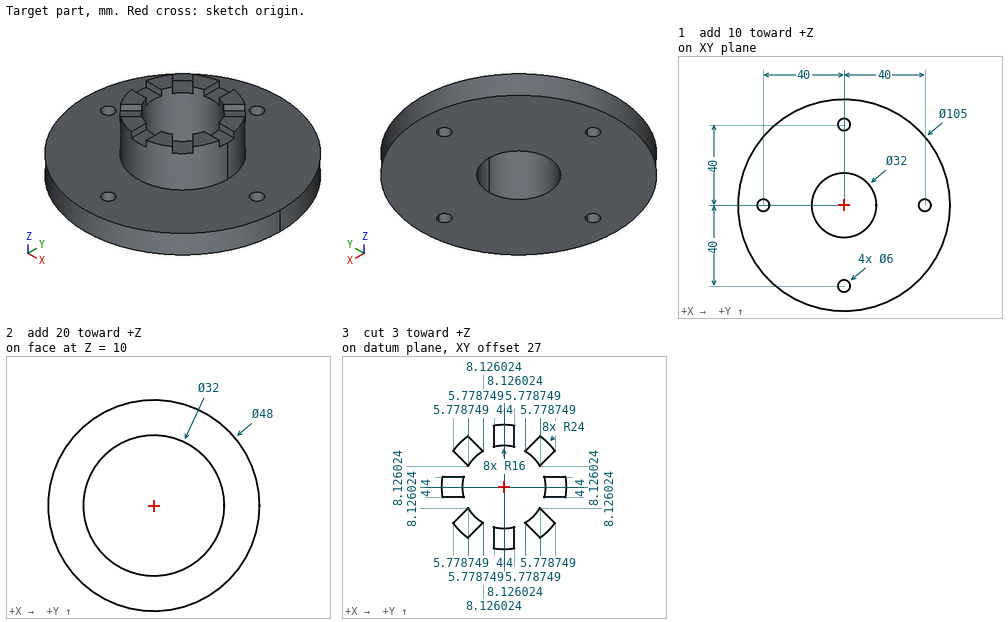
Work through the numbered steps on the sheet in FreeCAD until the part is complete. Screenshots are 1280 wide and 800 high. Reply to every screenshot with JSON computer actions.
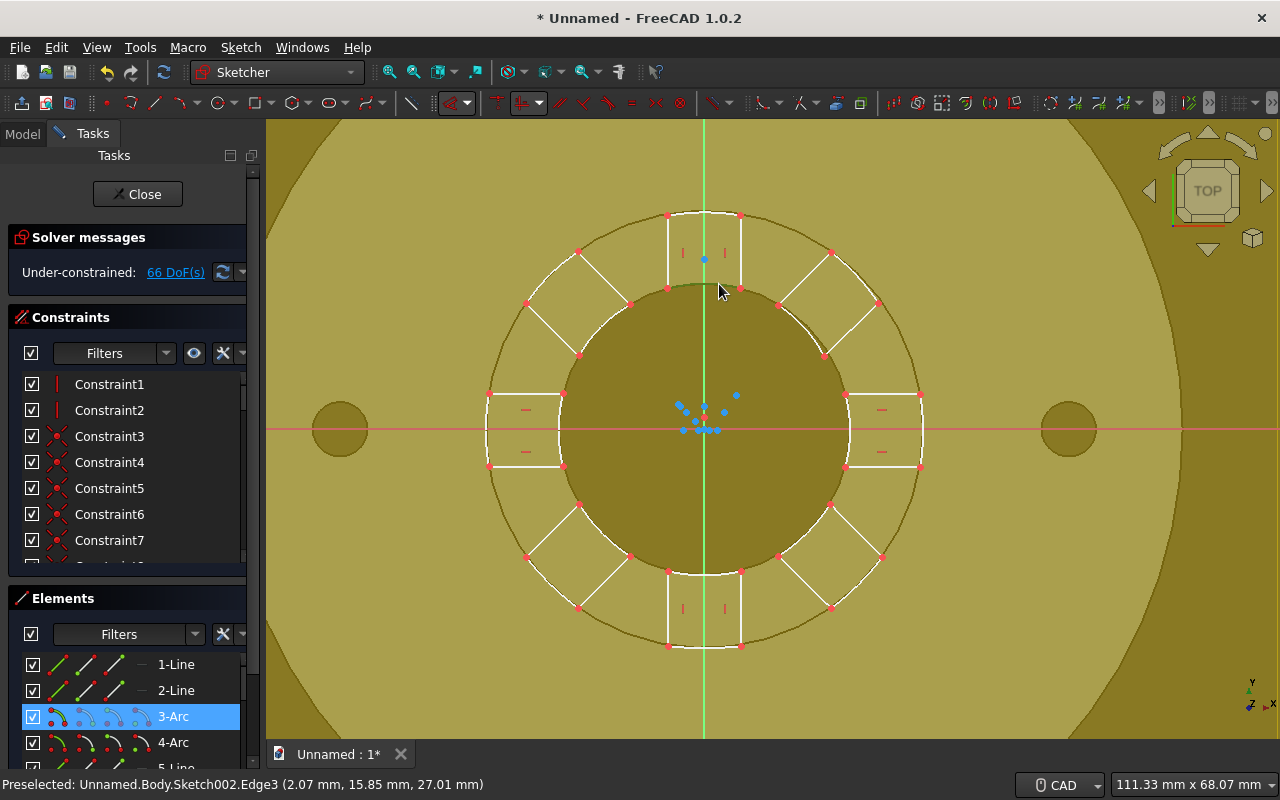
{"action": "left_click", "coordinate": [849, 445]}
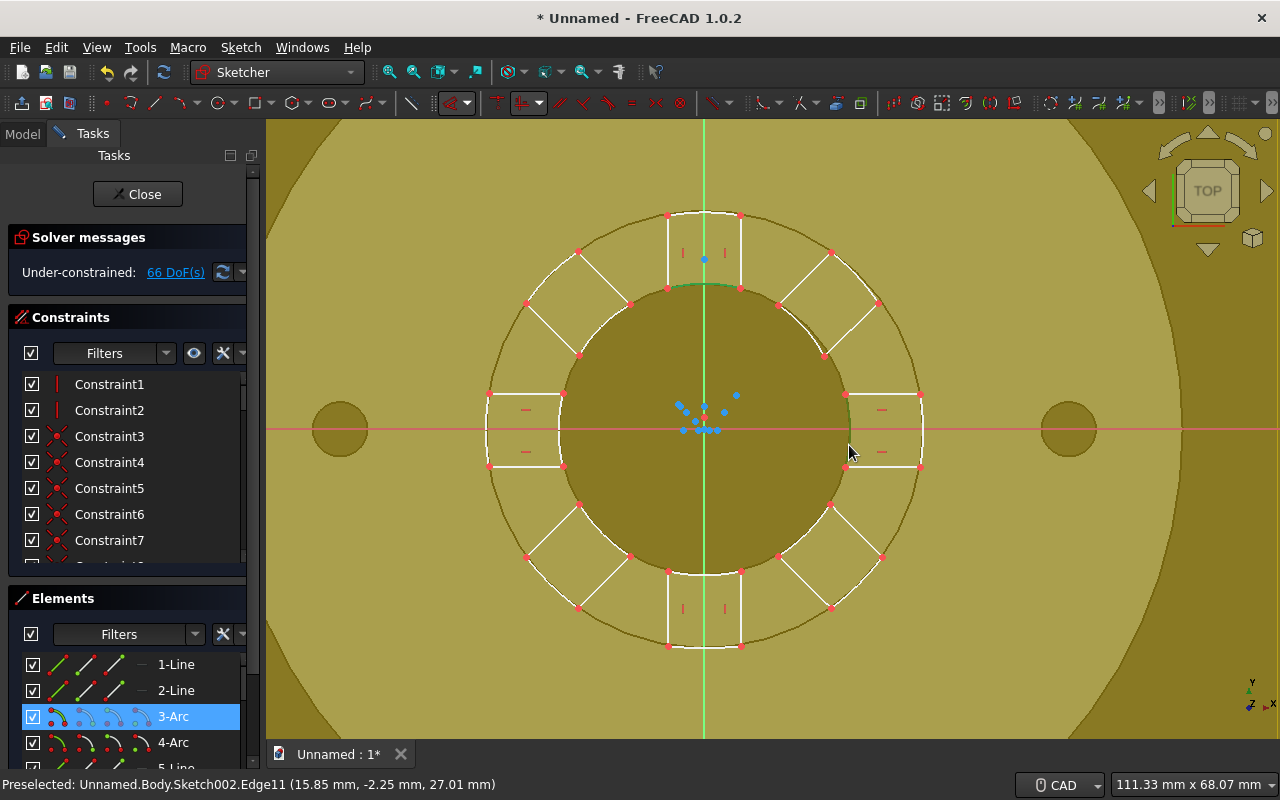
{"action": "left_click", "coordinate": [498, 104]}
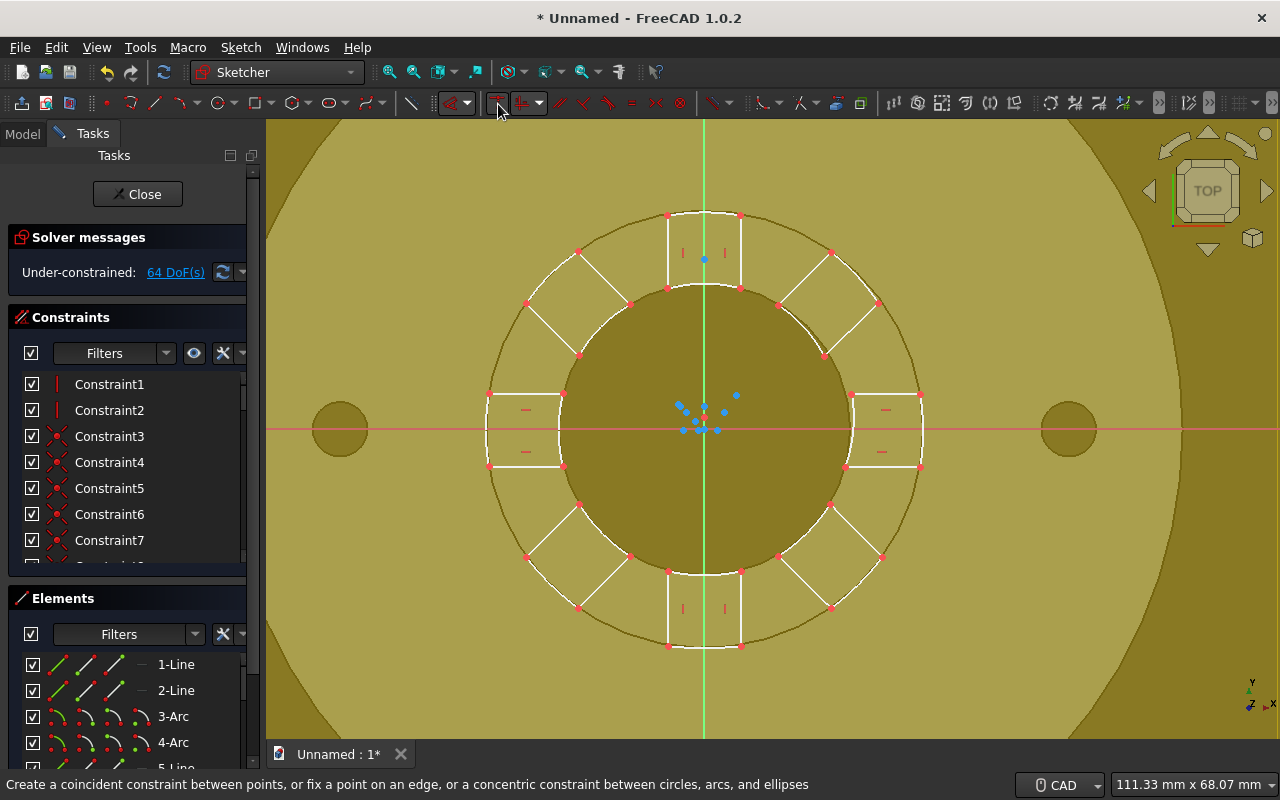
{"action": "left_click", "coordinate": [719, 284]}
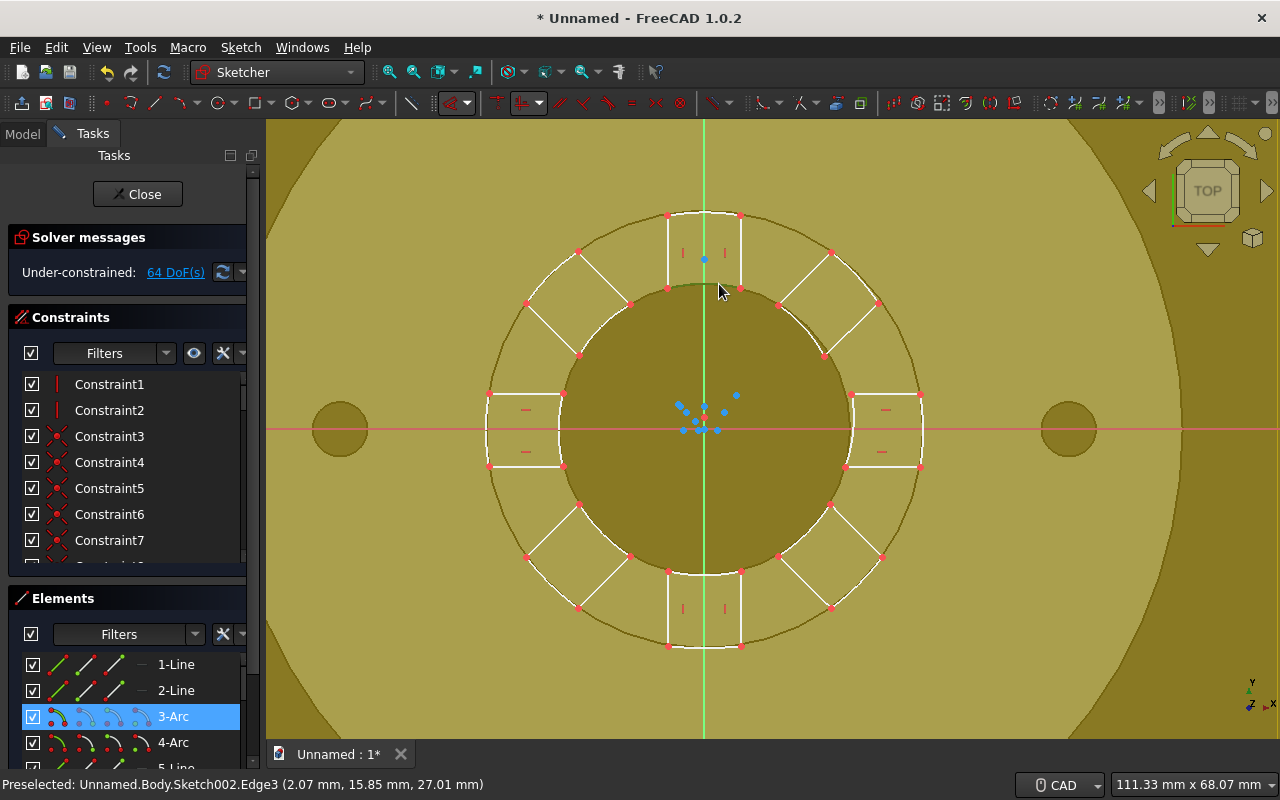
{"action": "left_click", "coordinate": [923, 445]}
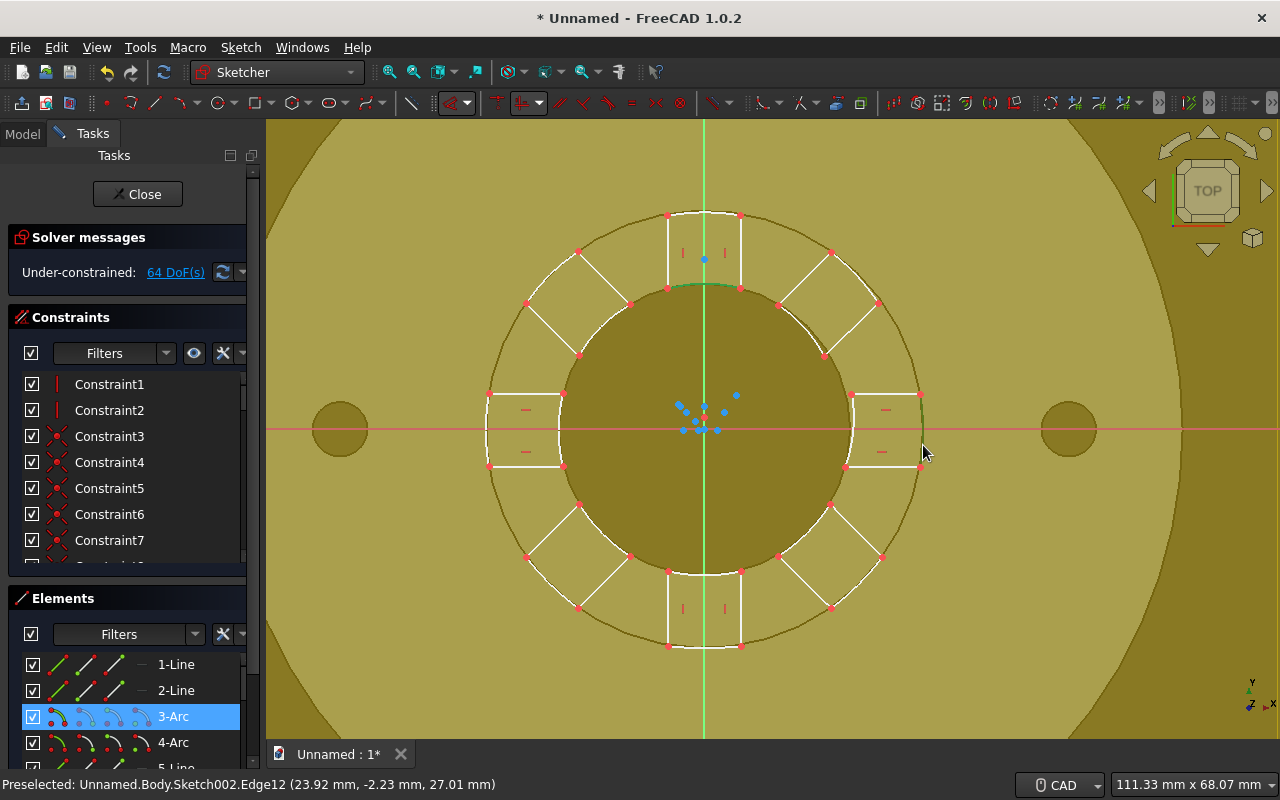
{"action": "left_click", "coordinate": [498, 104]}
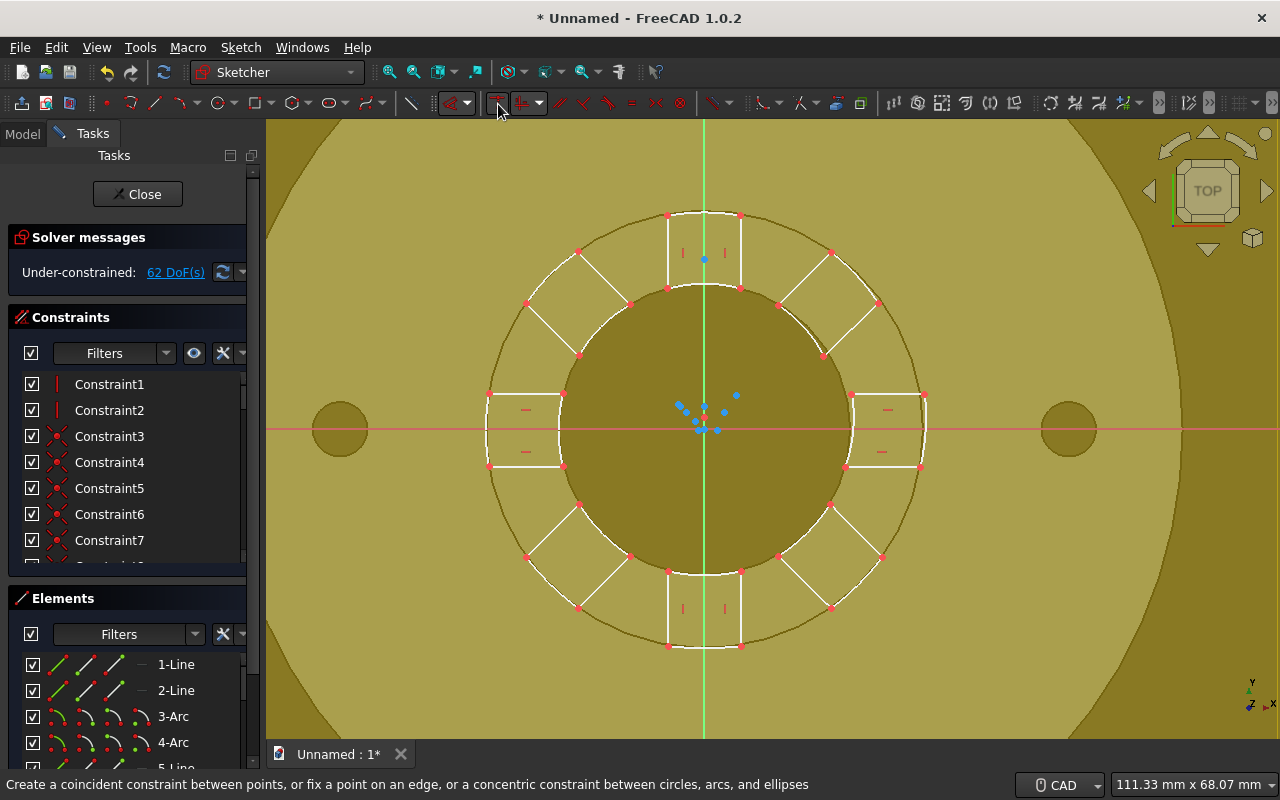
{"action": "left_click", "coordinate": [719, 285]}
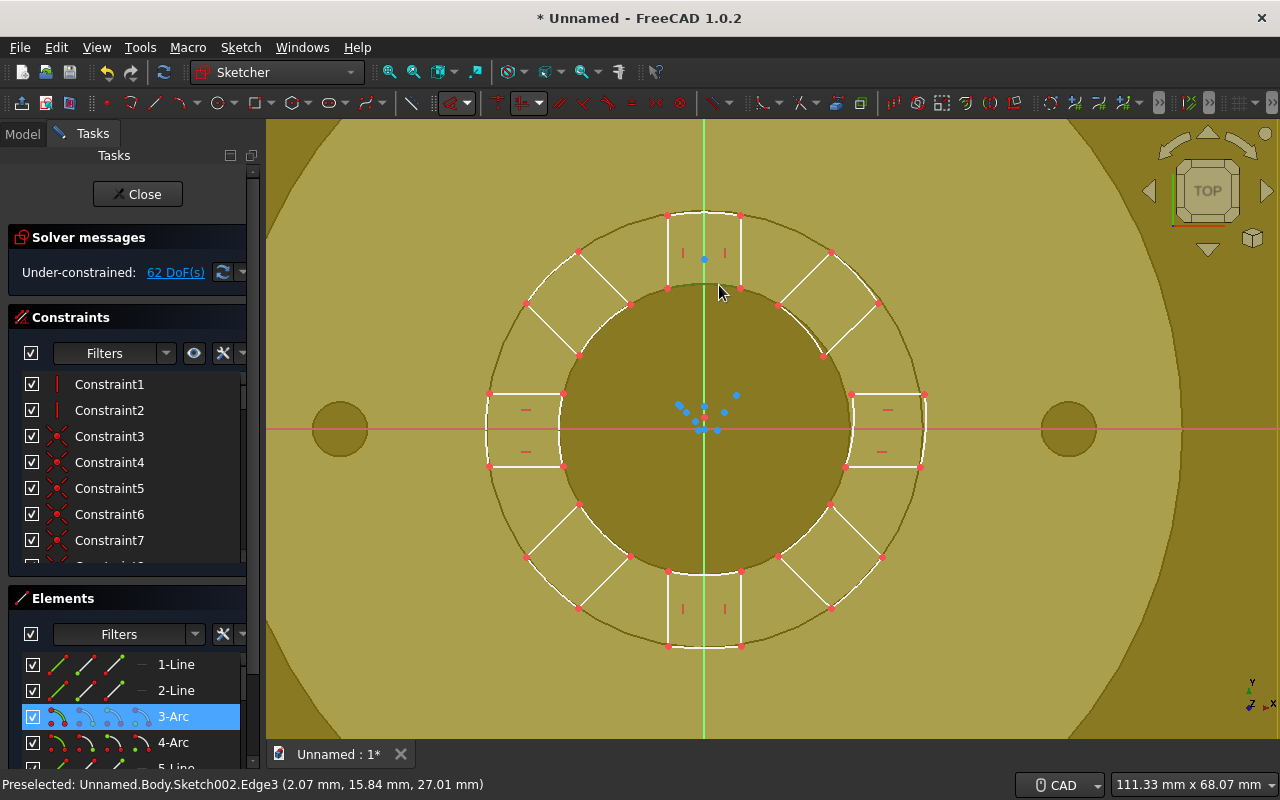
{"action": "left_click", "coordinate": [796, 543]}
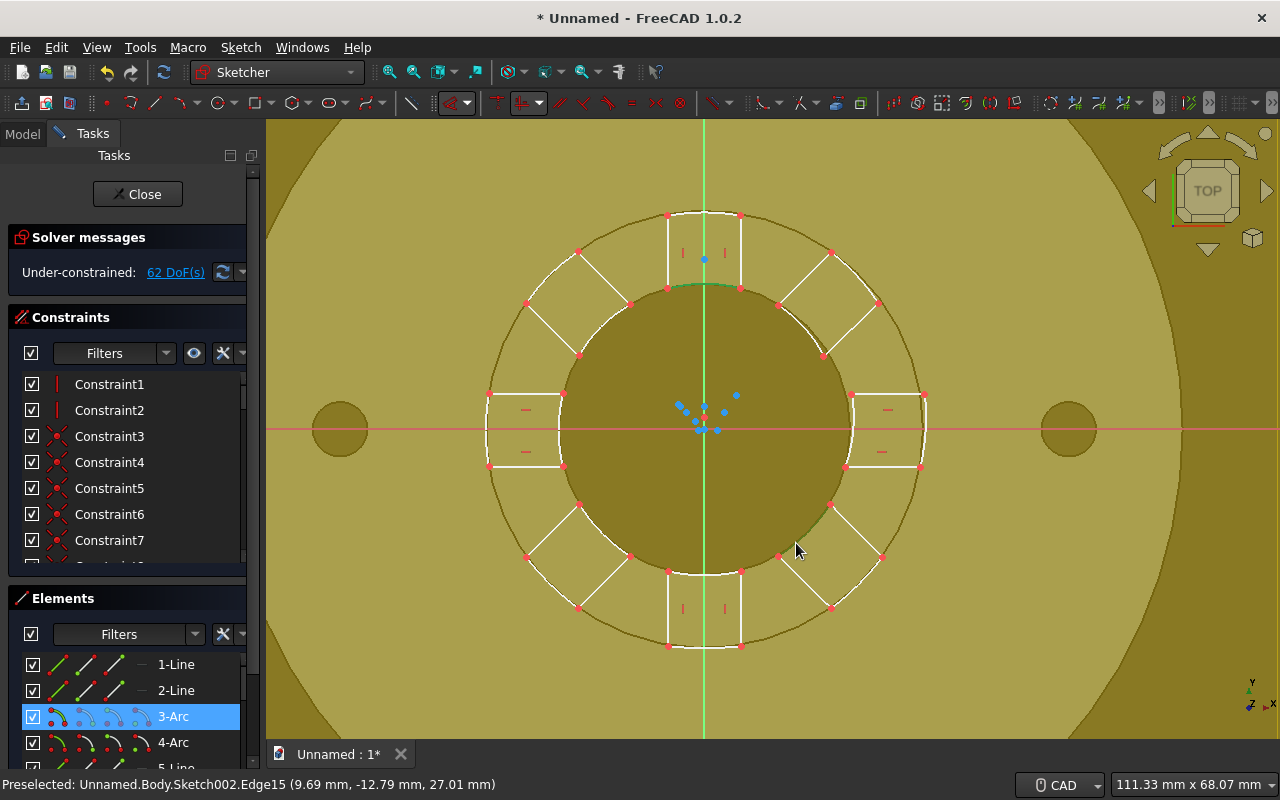
{"action": "left_click", "coordinate": [498, 104]}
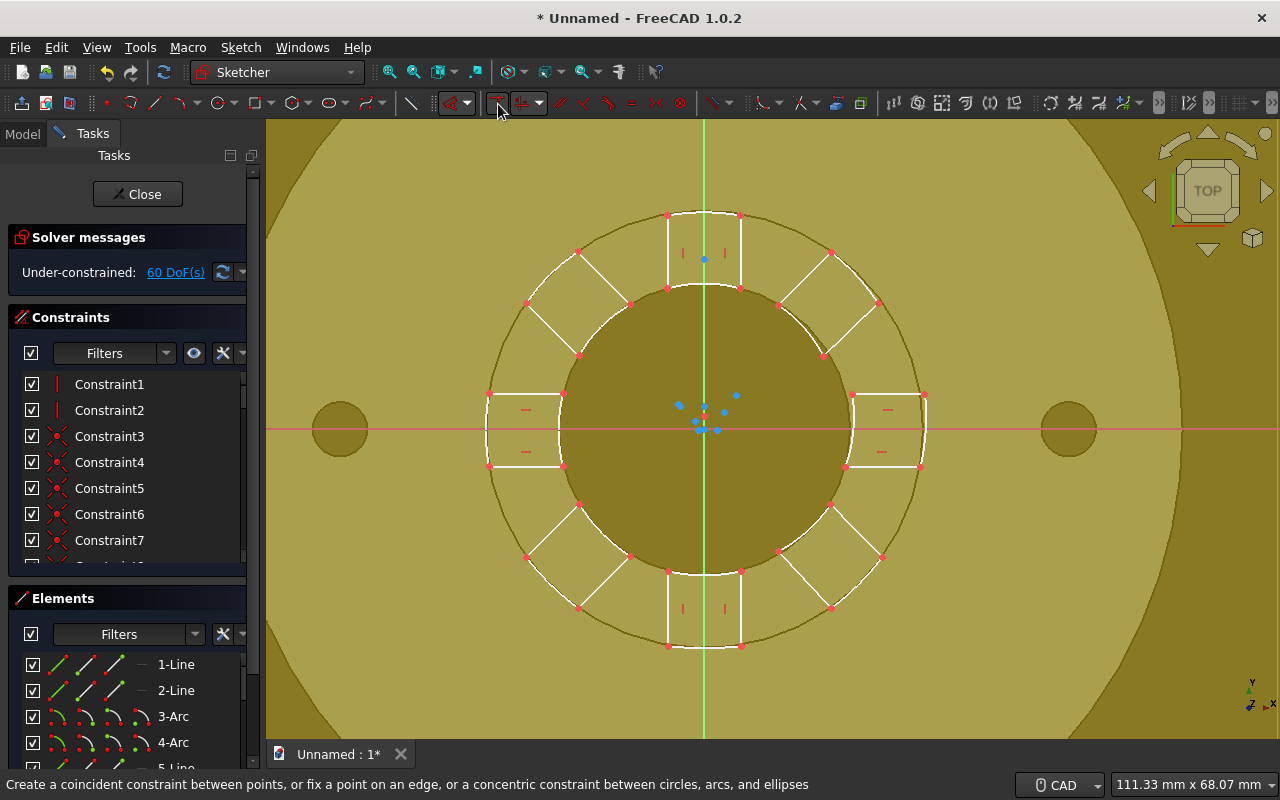
{"action": "left_click", "coordinate": [719, 284]}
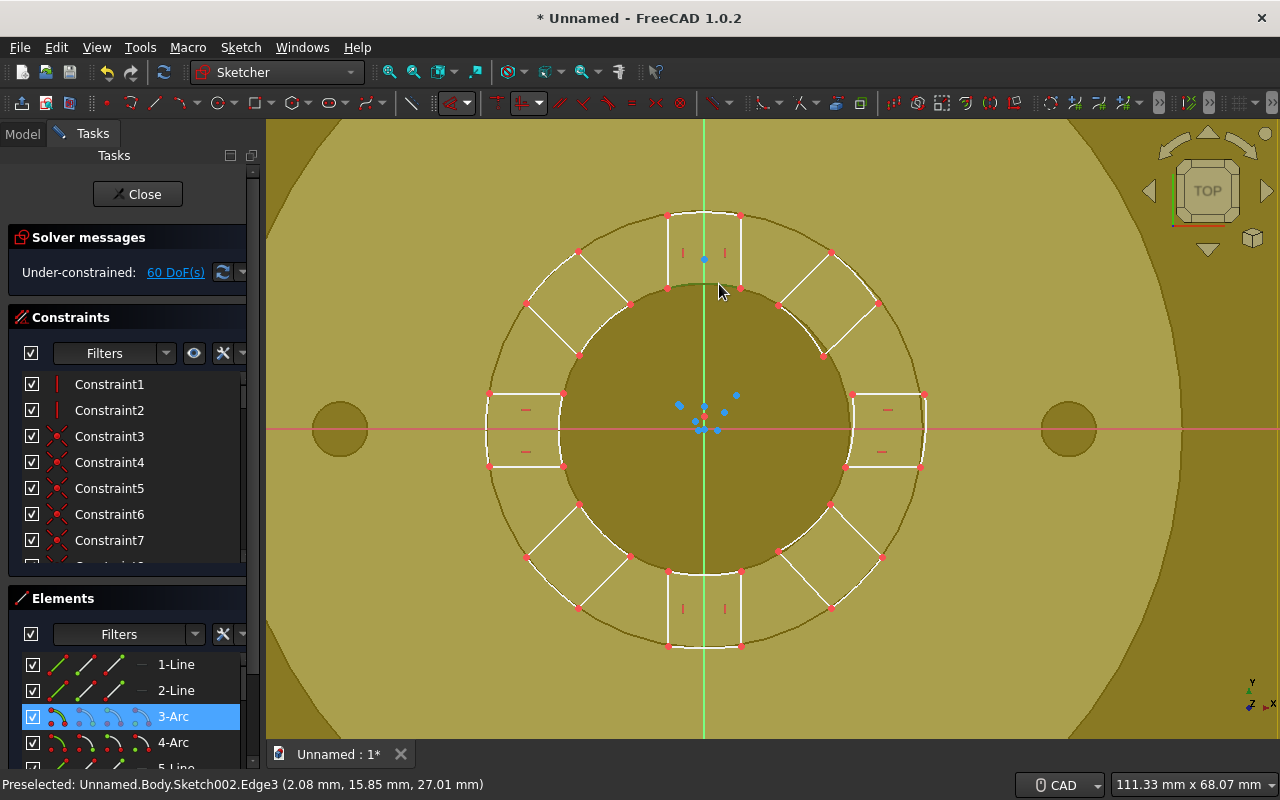
{"action": "left_click", "coordinate": [848, 594]}